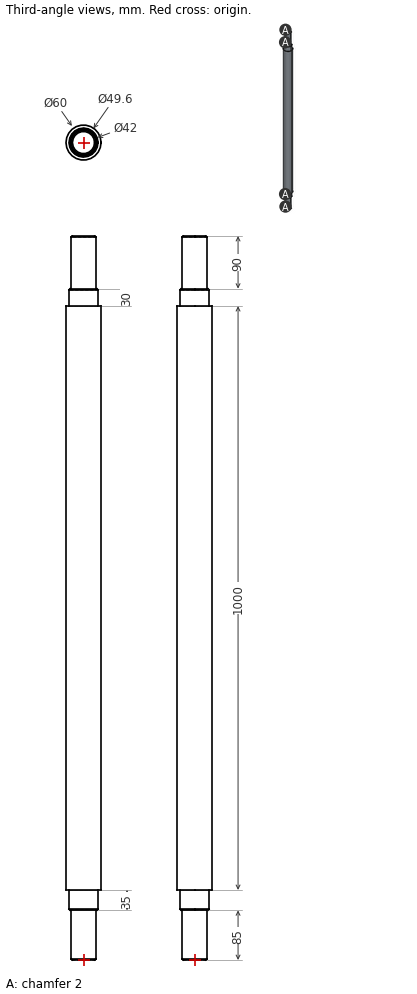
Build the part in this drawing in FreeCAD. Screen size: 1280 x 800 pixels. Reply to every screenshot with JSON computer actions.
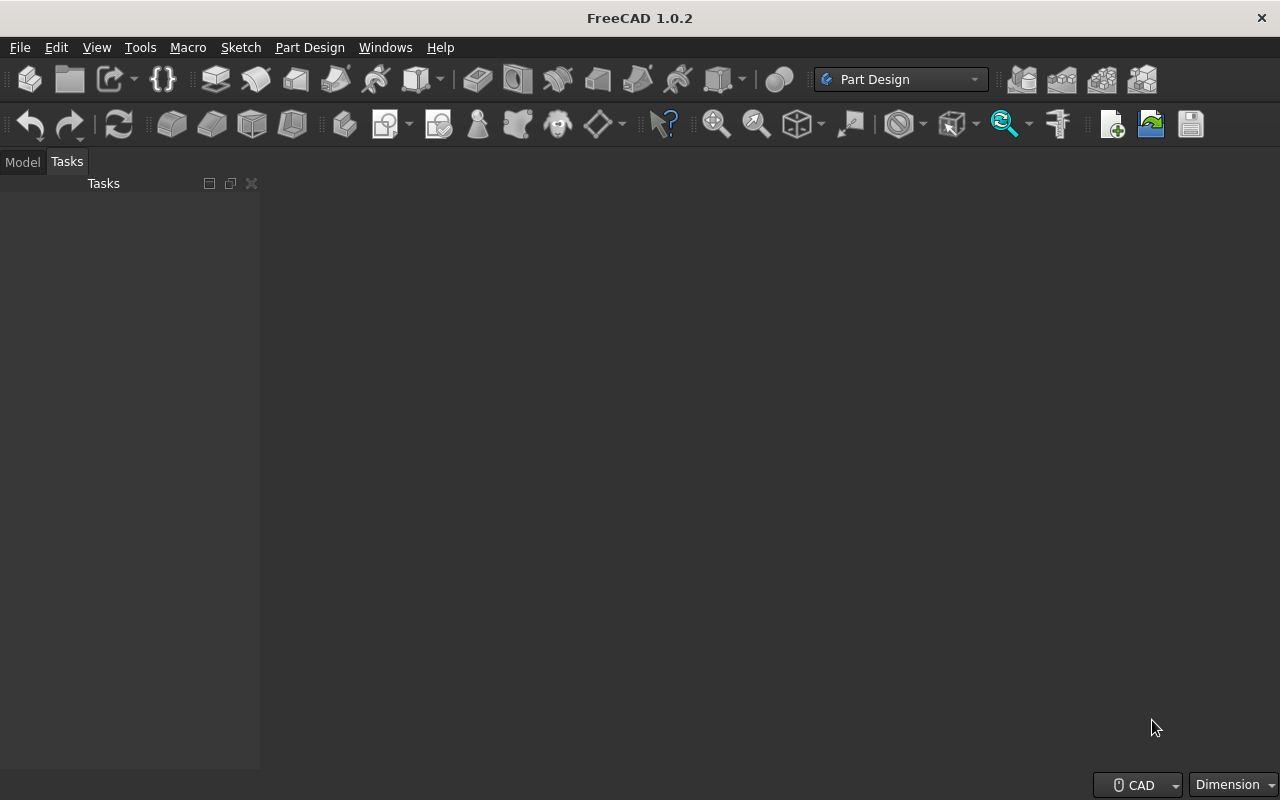
{"action": "key", "text": "ctrl+n"}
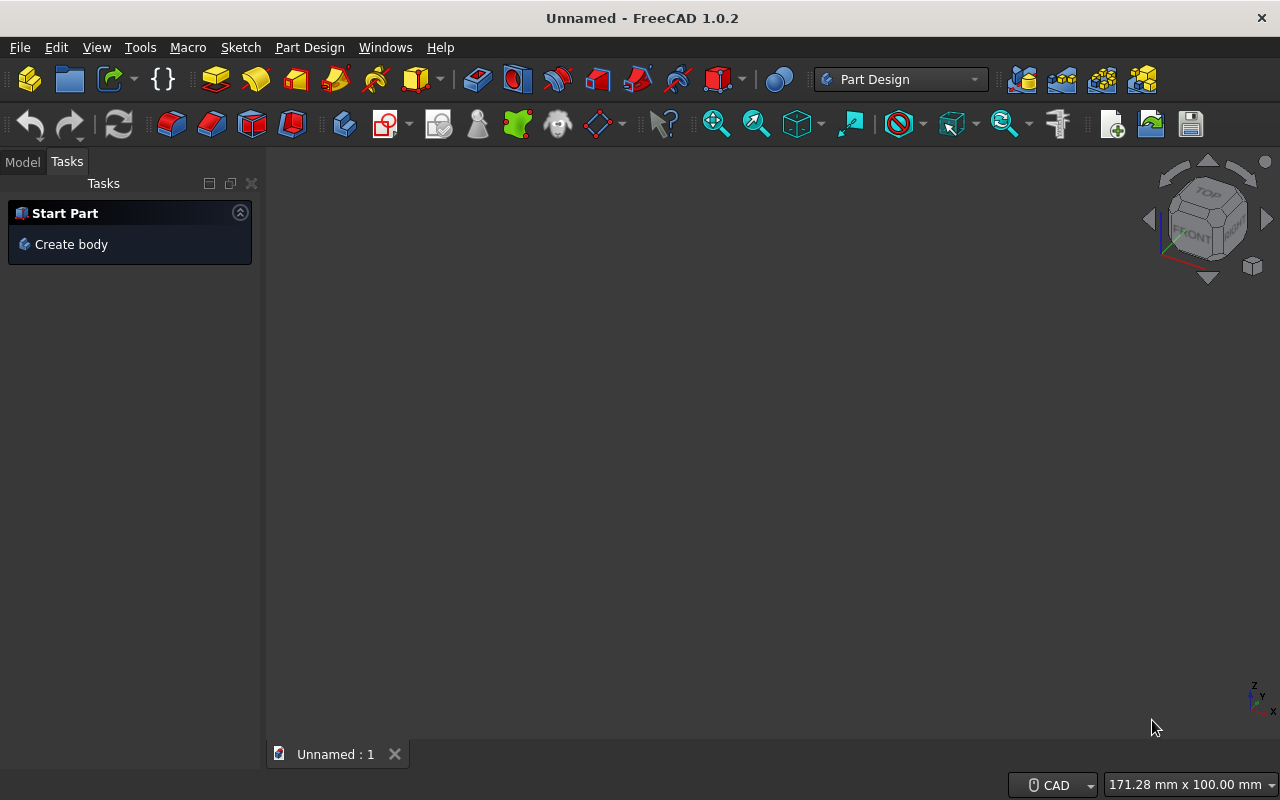
{"action": "left_click", "coordinate": [386, 124]}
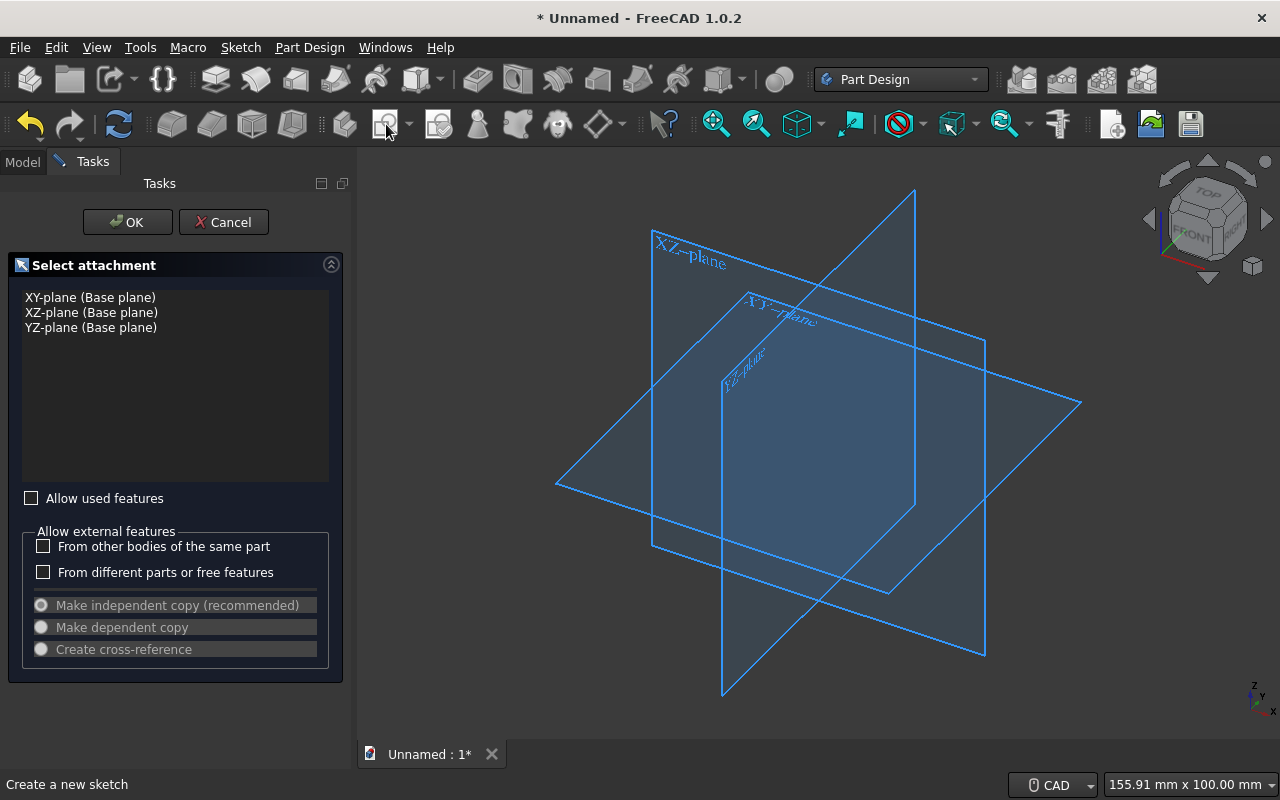
{"action": "left_click", "coordinate": [82, 298]}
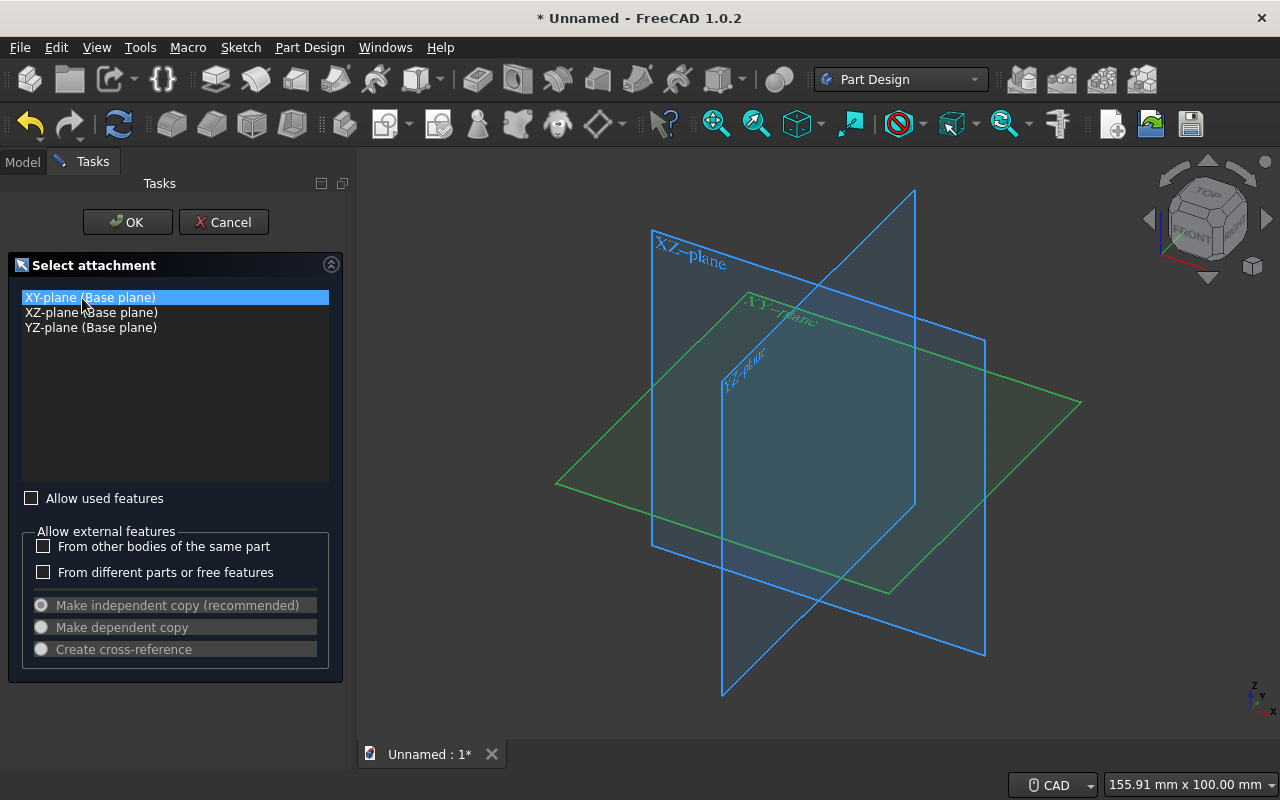
{"action": "left_click", "coordinate": [128, 222]}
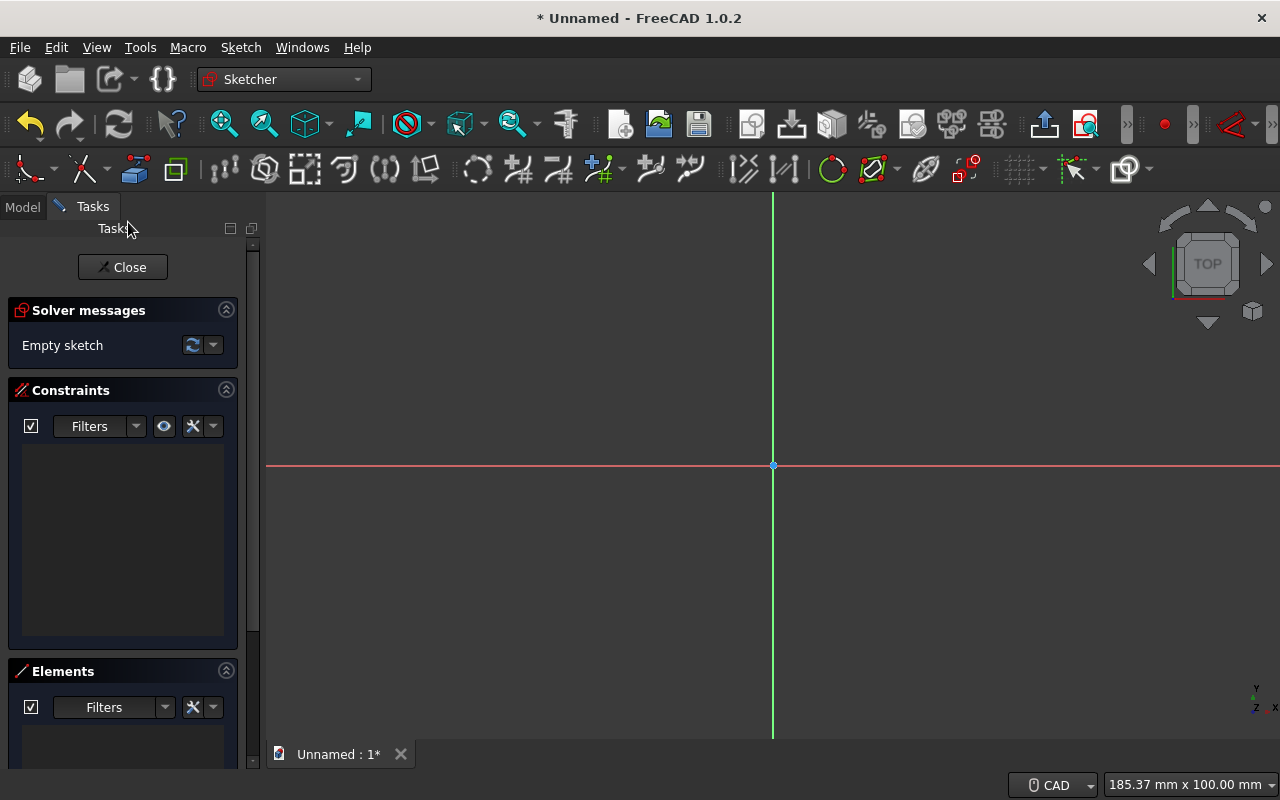
{"action": "scroll", "coordinate": [912, 466], "scroll_direction": "up", "scroll_amount": 2}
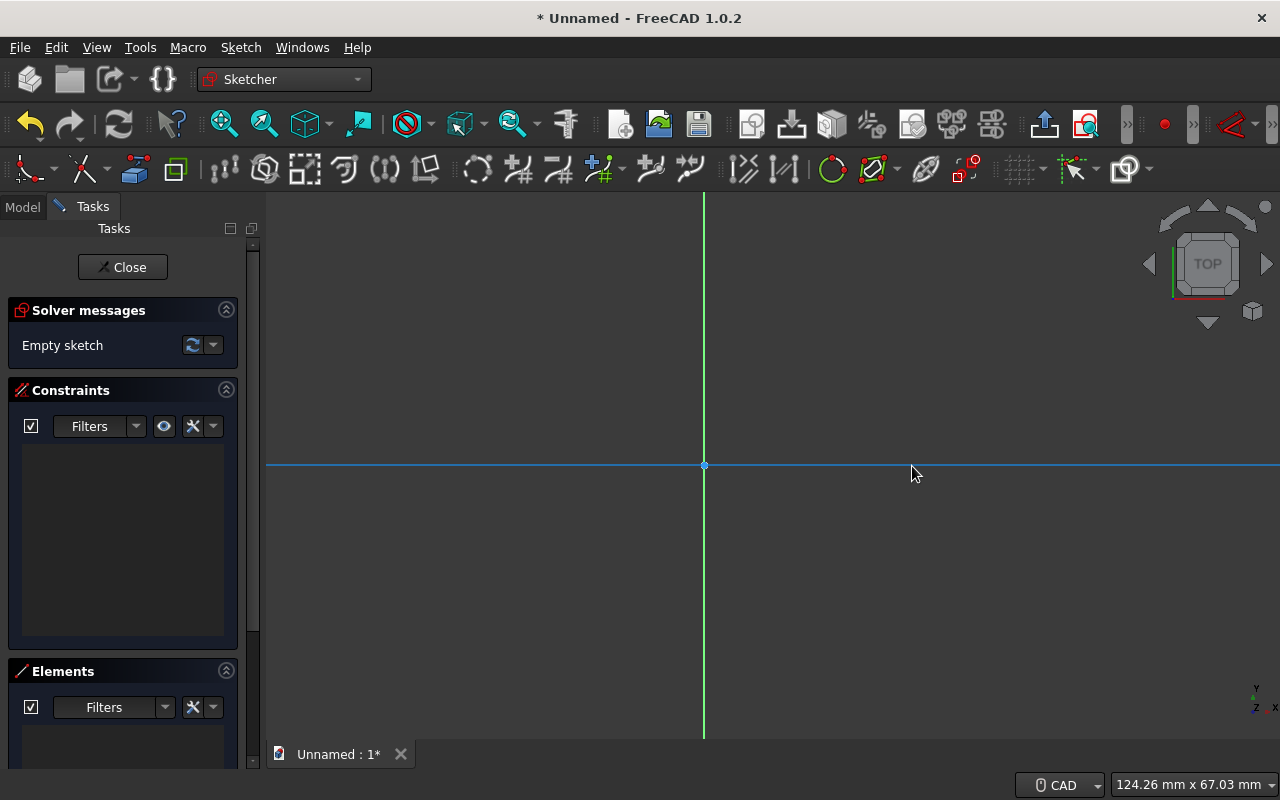
{"action": "key", "text": "g c"}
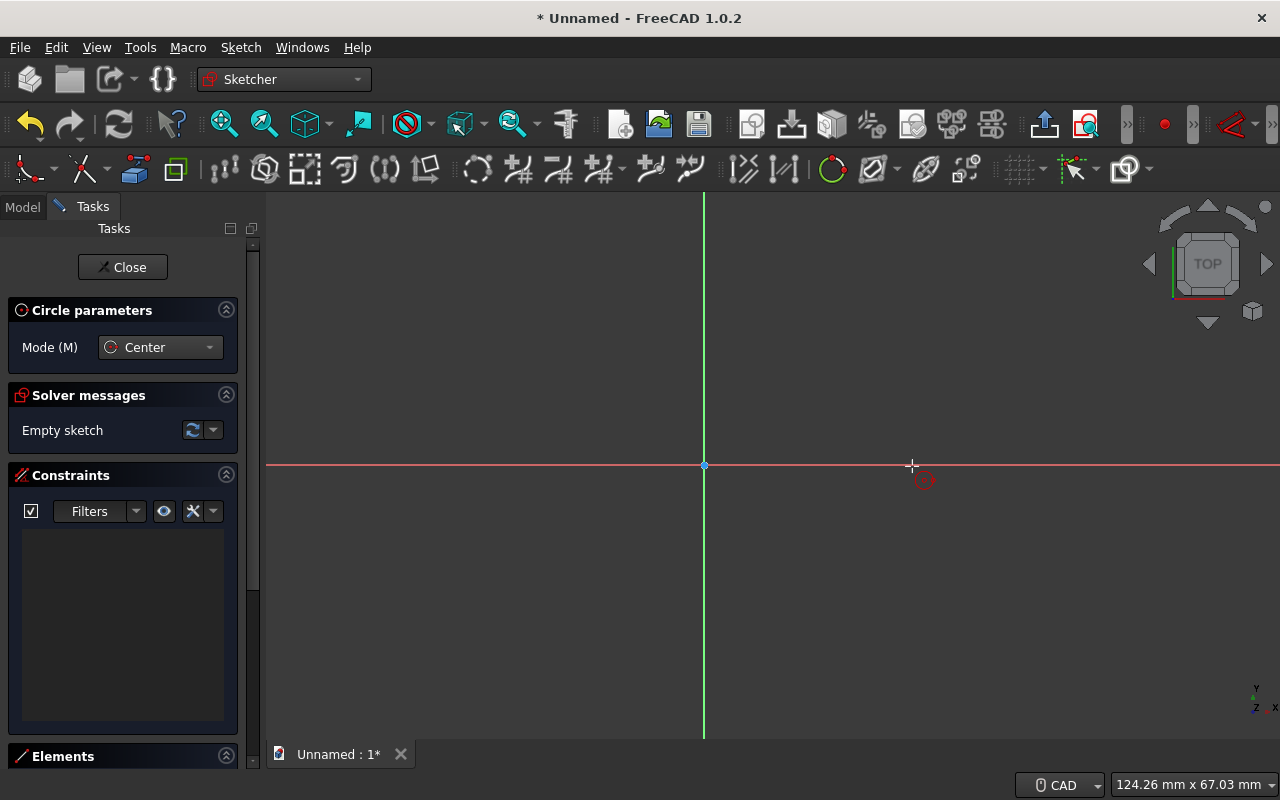
{"action": "left_click", "coordinate": [704, 465]}
{"action": "mouse_move", "coordinate": [825, 344]}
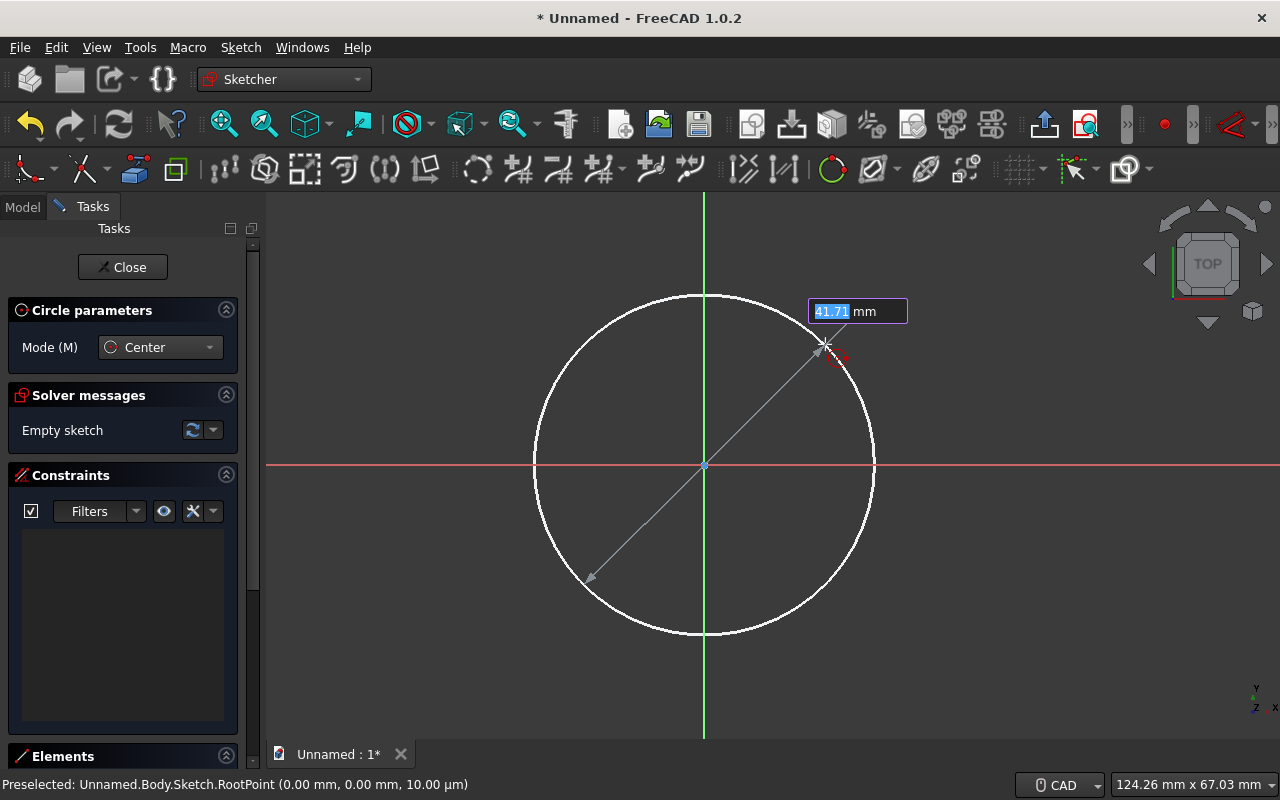
{"action": "type", "text": "42"}
{"action": "key", "text": "Return"}
{"action": "key", "text": "Escape"}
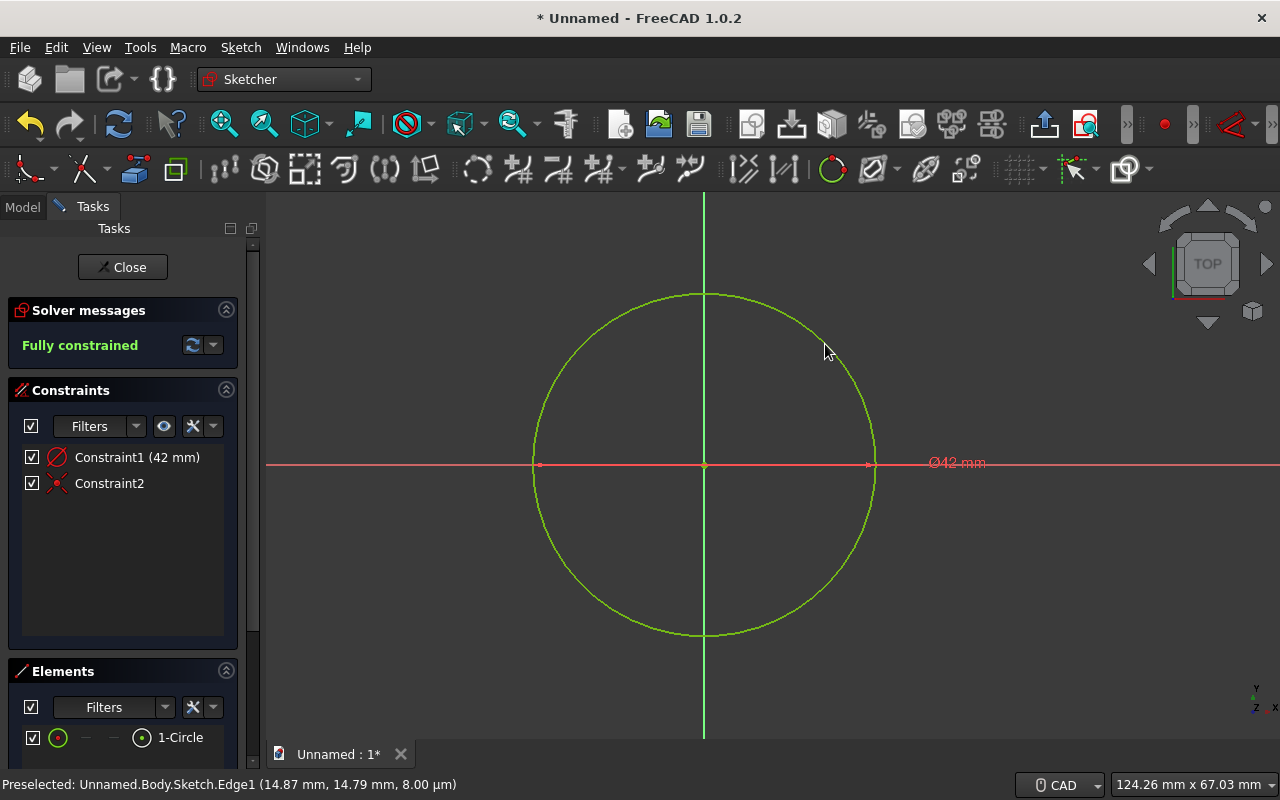
{"action": "left_click", "coordinate": [123, 267]}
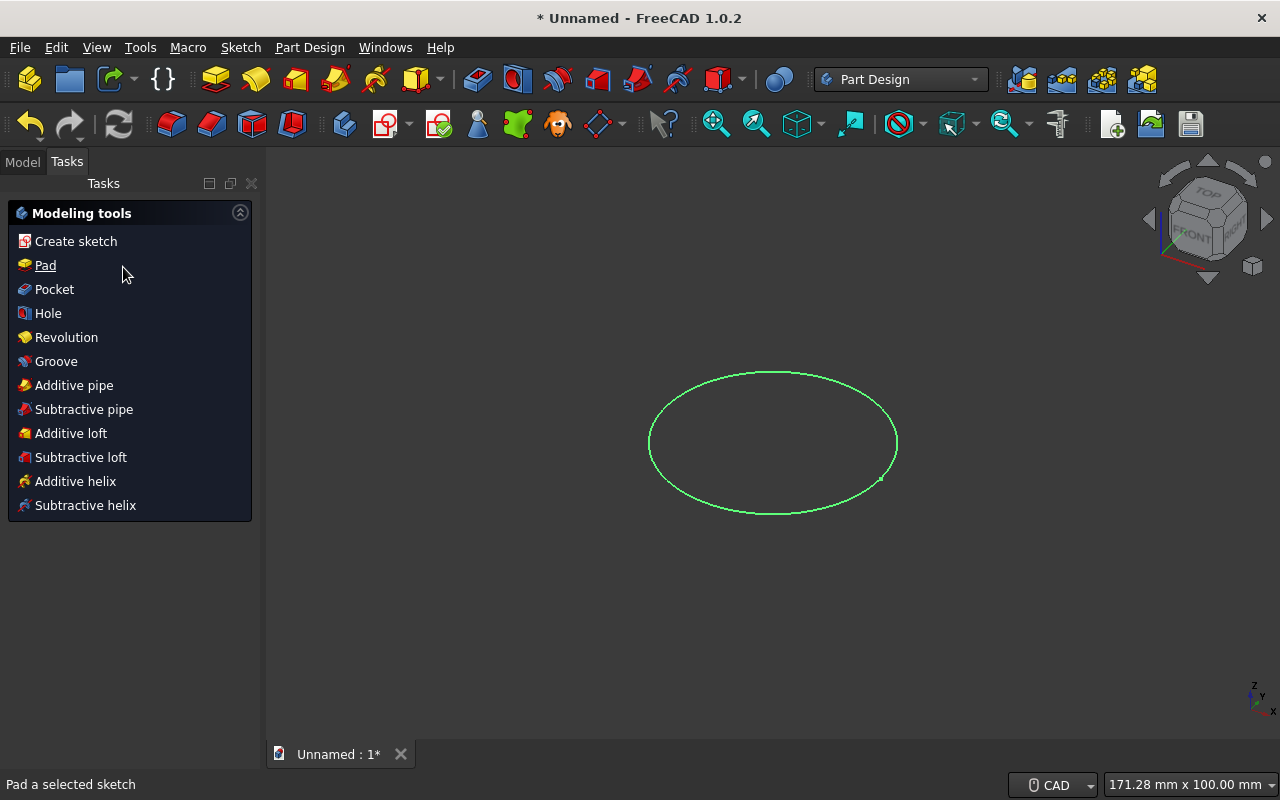
{"action": "left_click", "coordinate": [216, 80]}